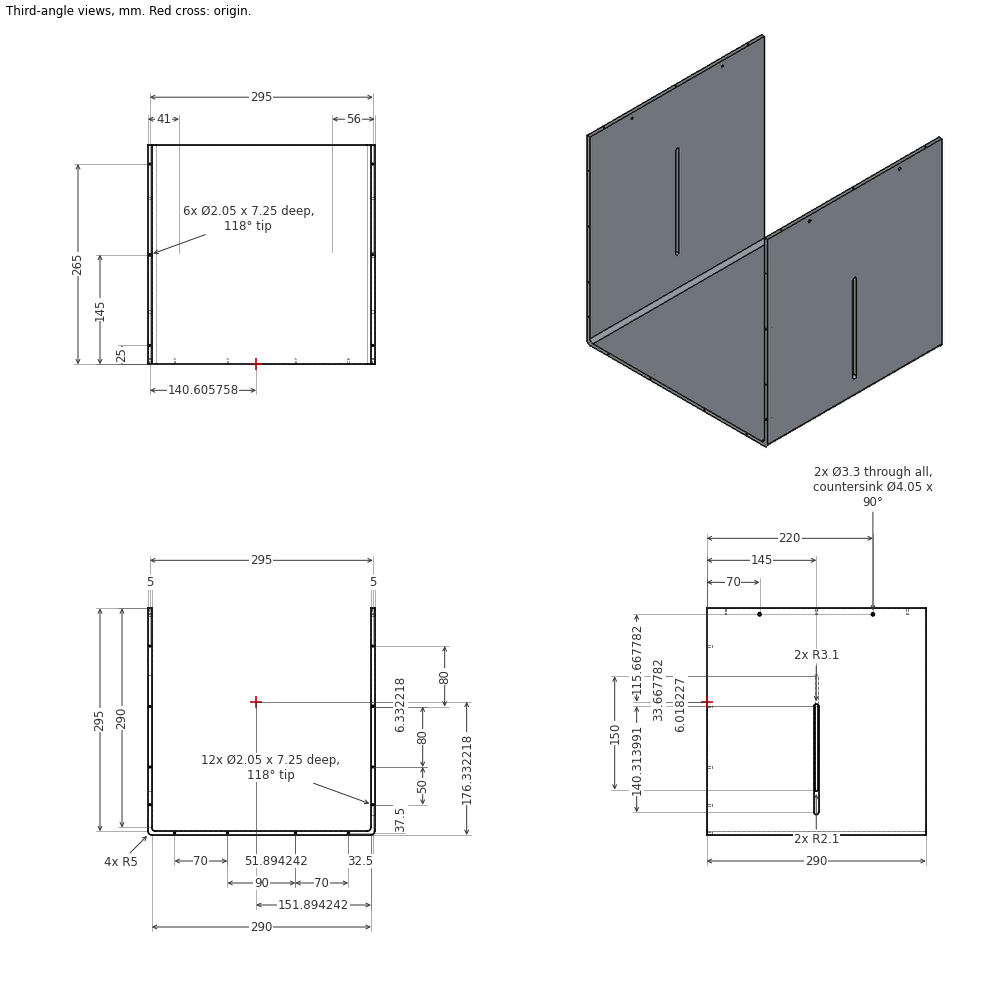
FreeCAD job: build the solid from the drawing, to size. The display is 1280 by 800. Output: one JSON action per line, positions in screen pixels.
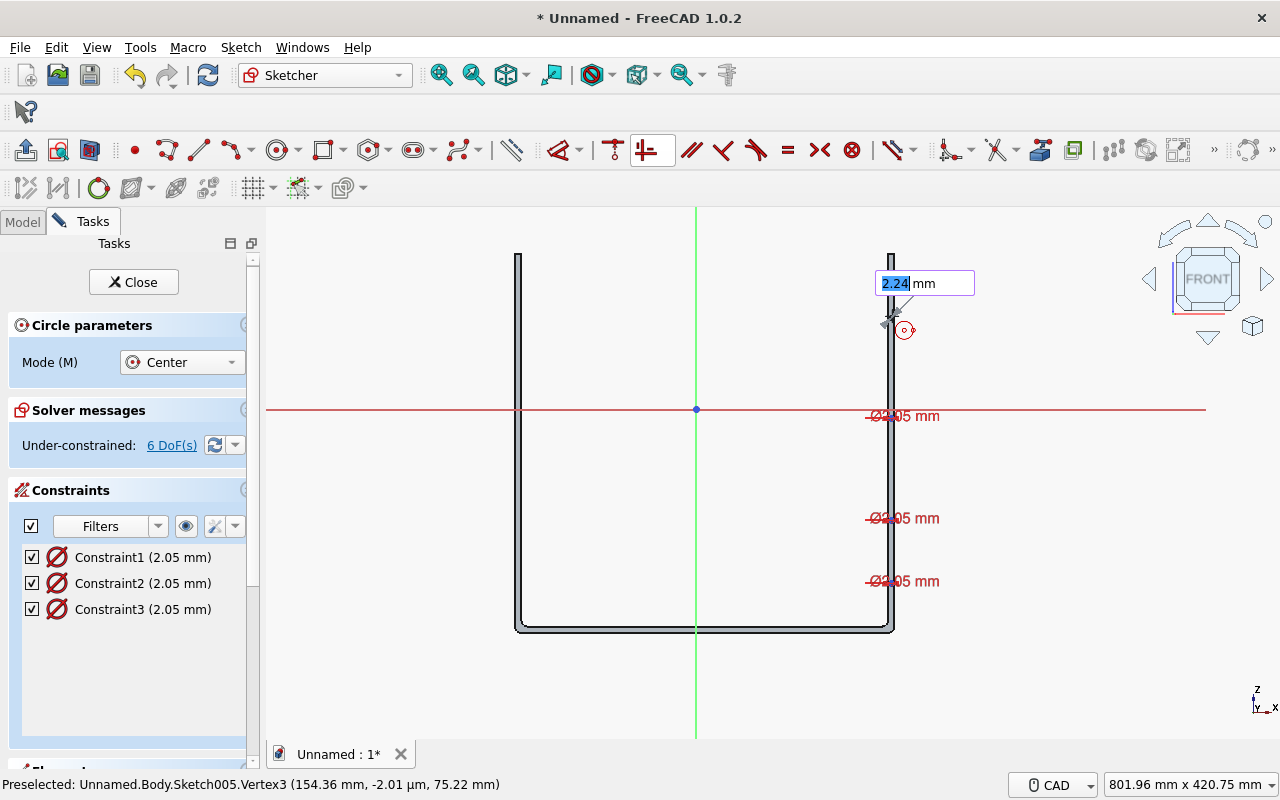
{"action": "type", "text": "2.05"}
{"action": "key", "text": "Return"}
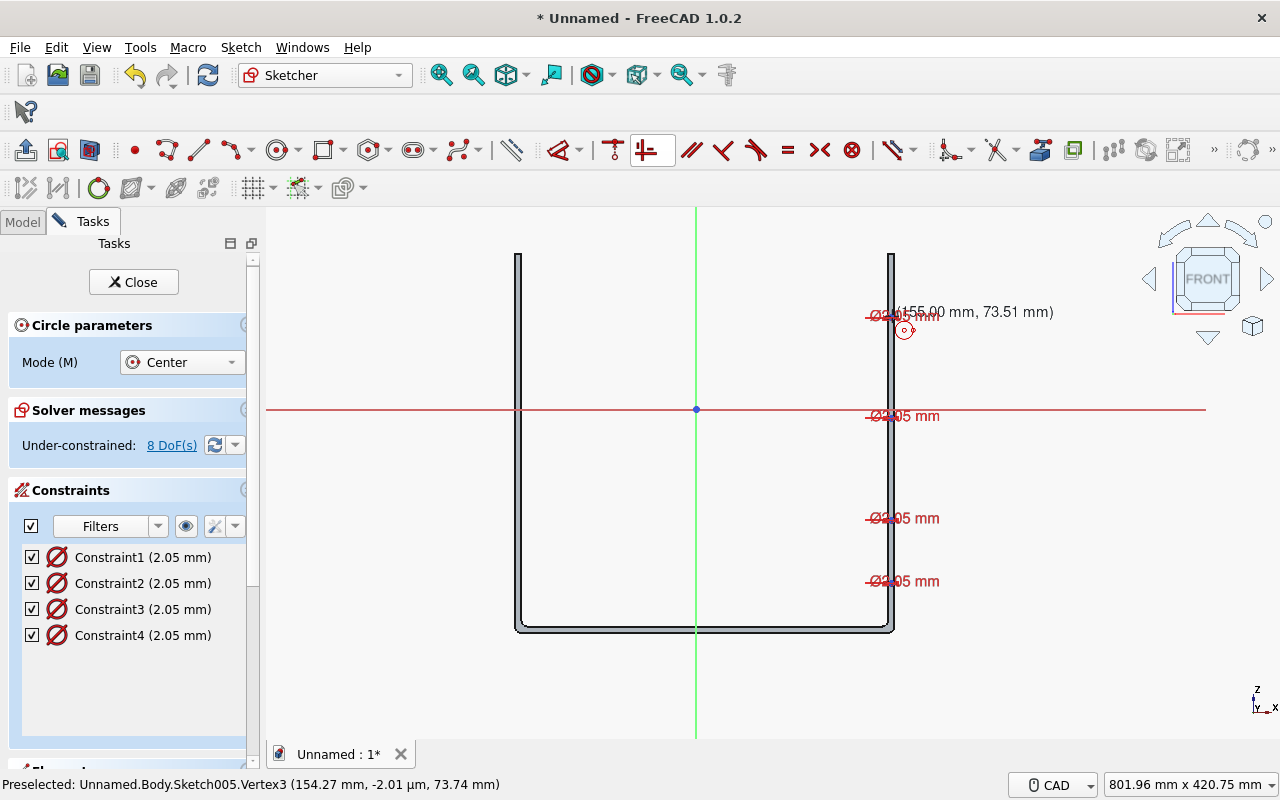
{"action": "scroll", "coordinate": [850, 630], "scroll_direction": "up", "scroll_amount": 15}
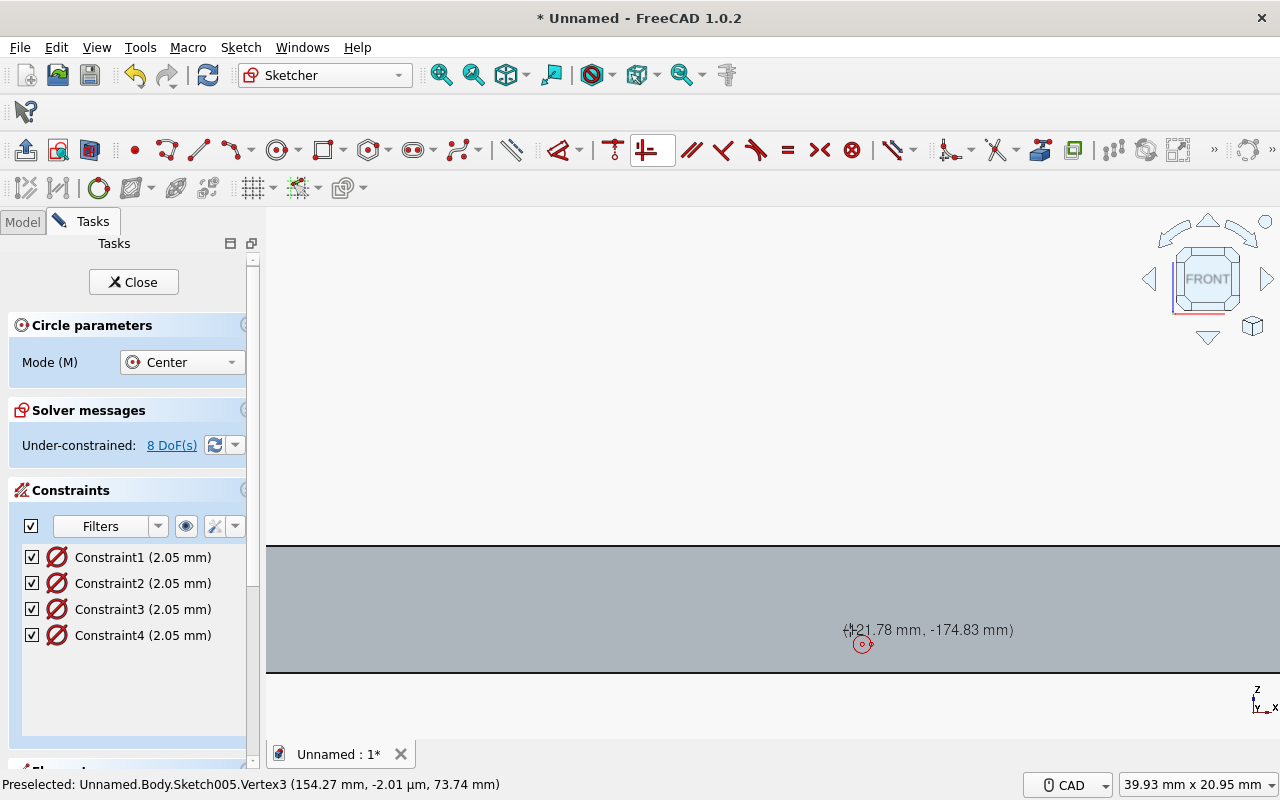
{"action": "scroll", "coordinate": [850, 631], "scroll_direction": "down", "scroll_amount": 15}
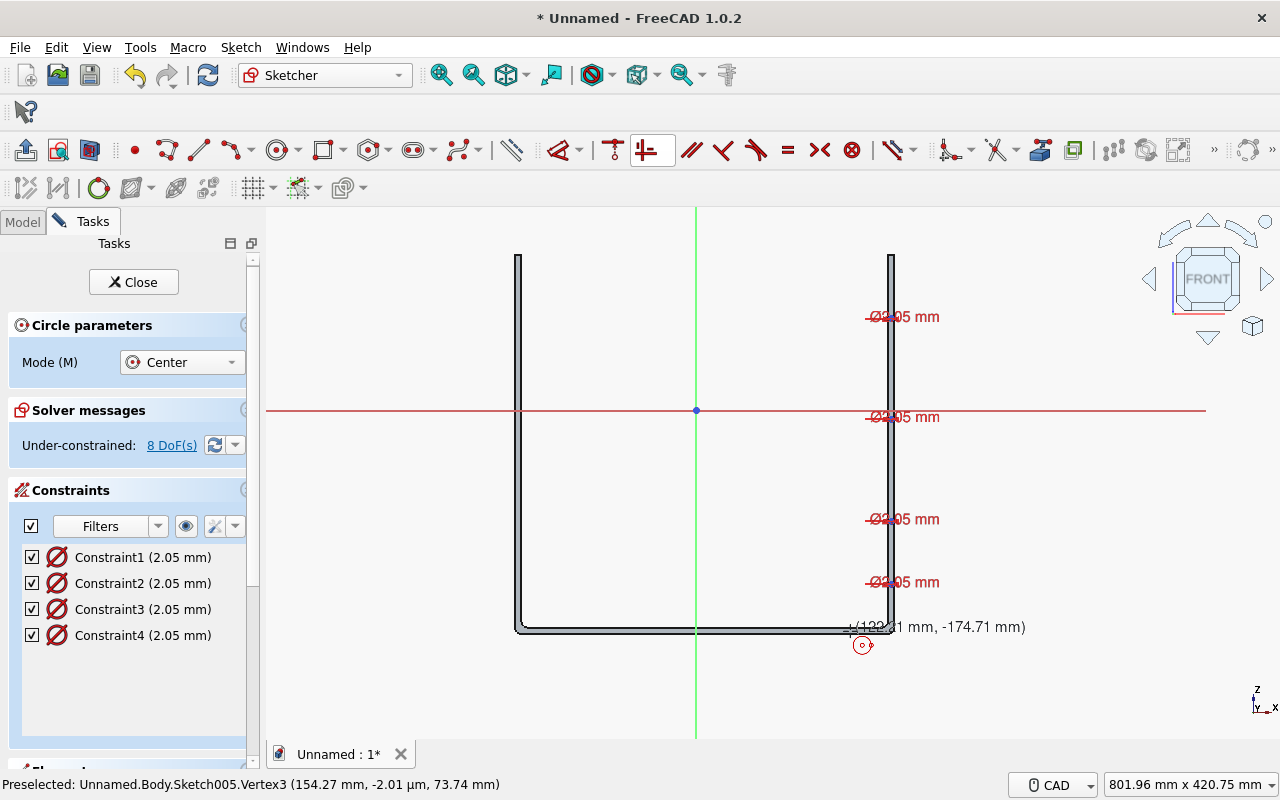
{"action": "left_click", "coordinate": [850, 631]}
{"action": "mouse_move", "coordinate": [851, 630]}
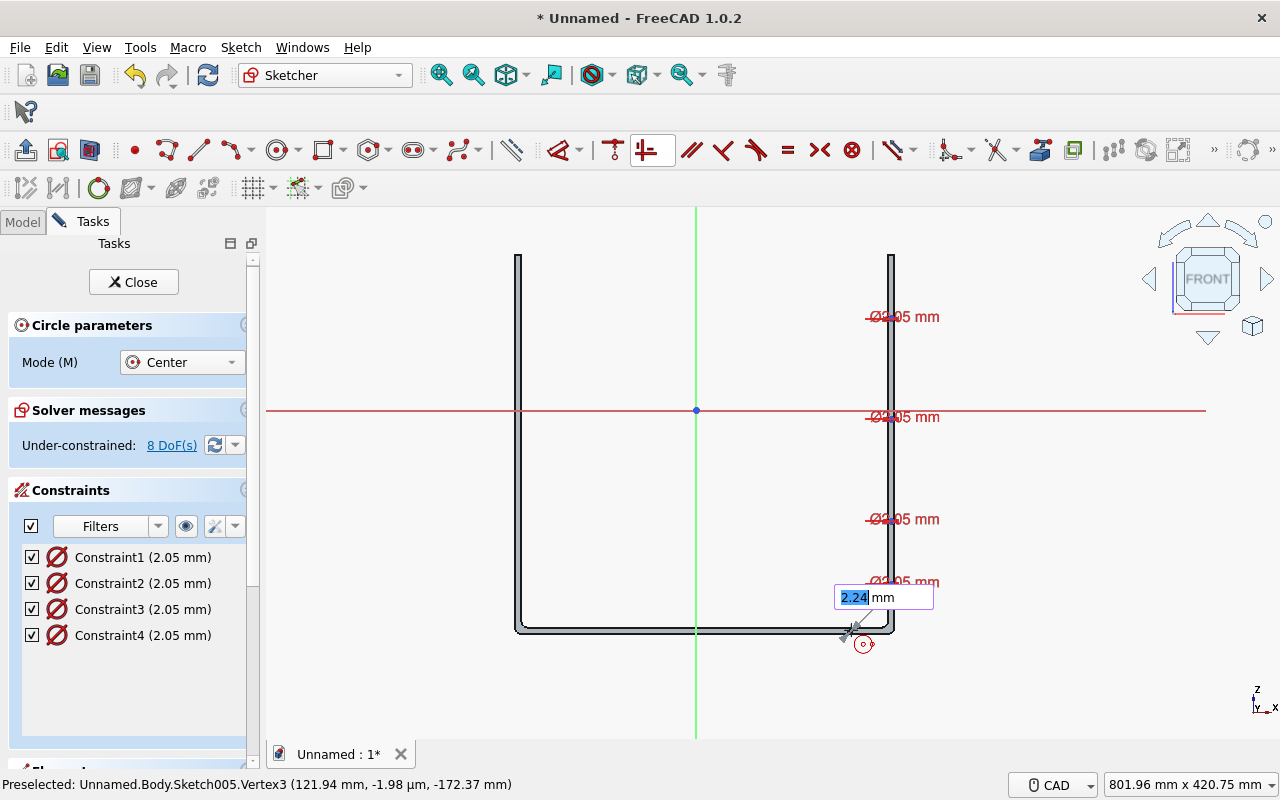
{"action": "type", "text": "2.05"}
{"action": "key", "text": "Return"}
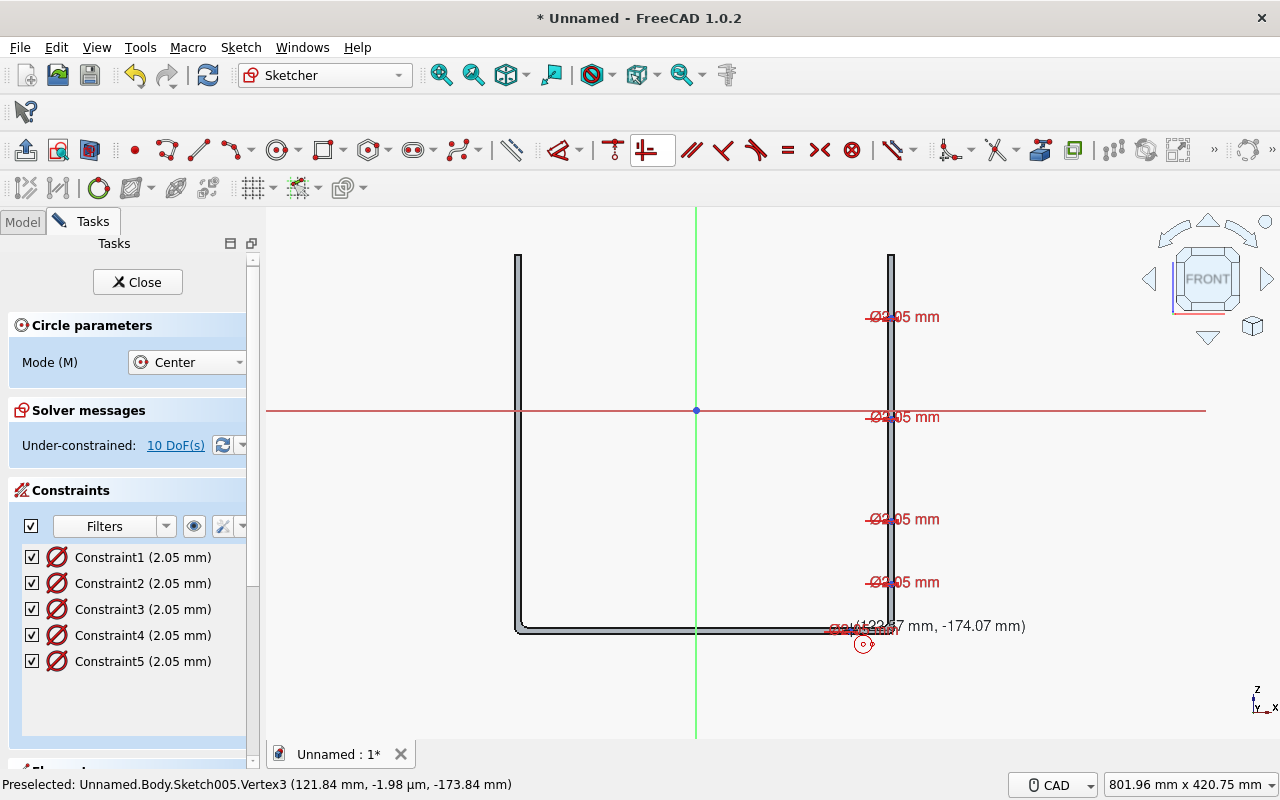
{"action": "scroll", "coordinate": [762, 631], "scroll_direction": "up", "scroll_amount": 15}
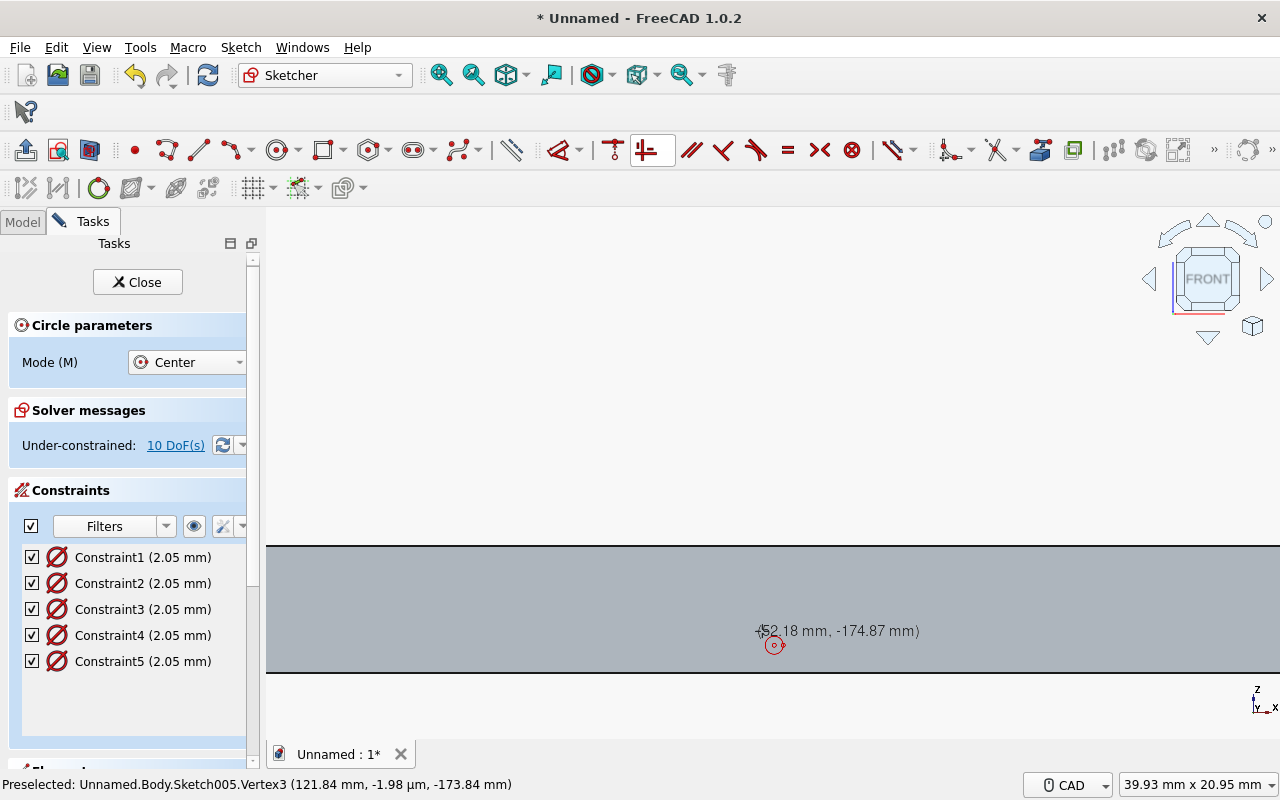
{"action": "scroll", "coordinate": [762, 631], "scroll_direction": "down", "scroll_amount": 15}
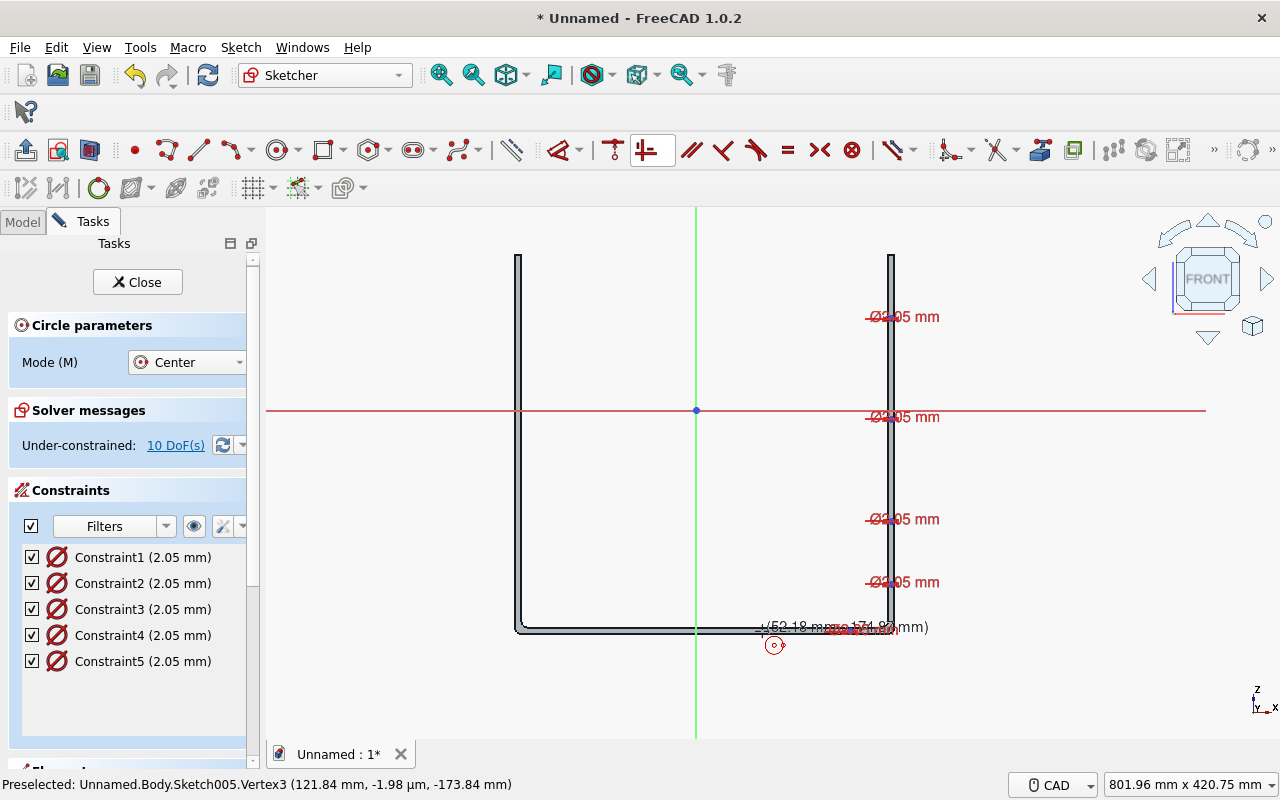
{"action": "left_click", "coordinate": [762, 631]}
{"action": "mouse_move", "coordinate": [763, 630]}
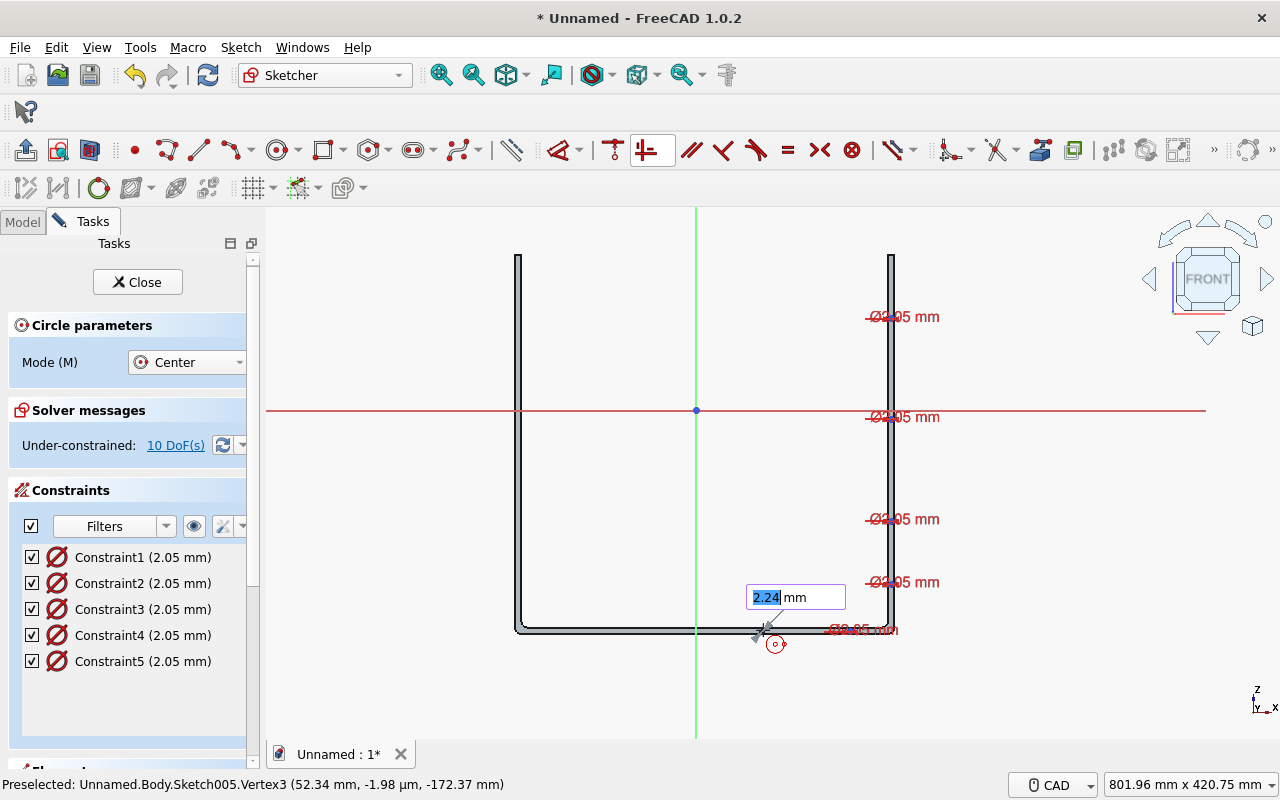
{"action": "type", "text": "2.05"}
{"action": "key", "text": "Return"}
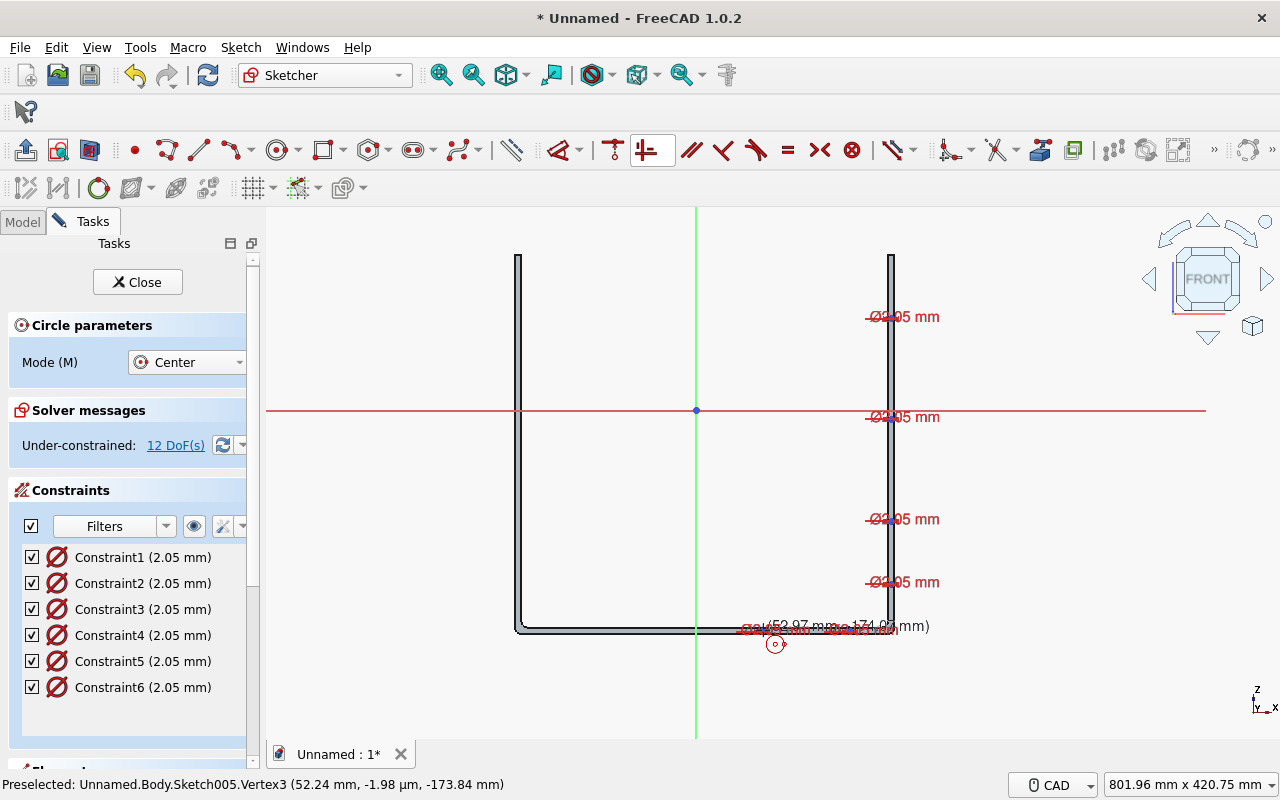
{"action": "scroll", "coordinate": [648, 631], "scroll_direction": "up", "scroll_amount": 15}